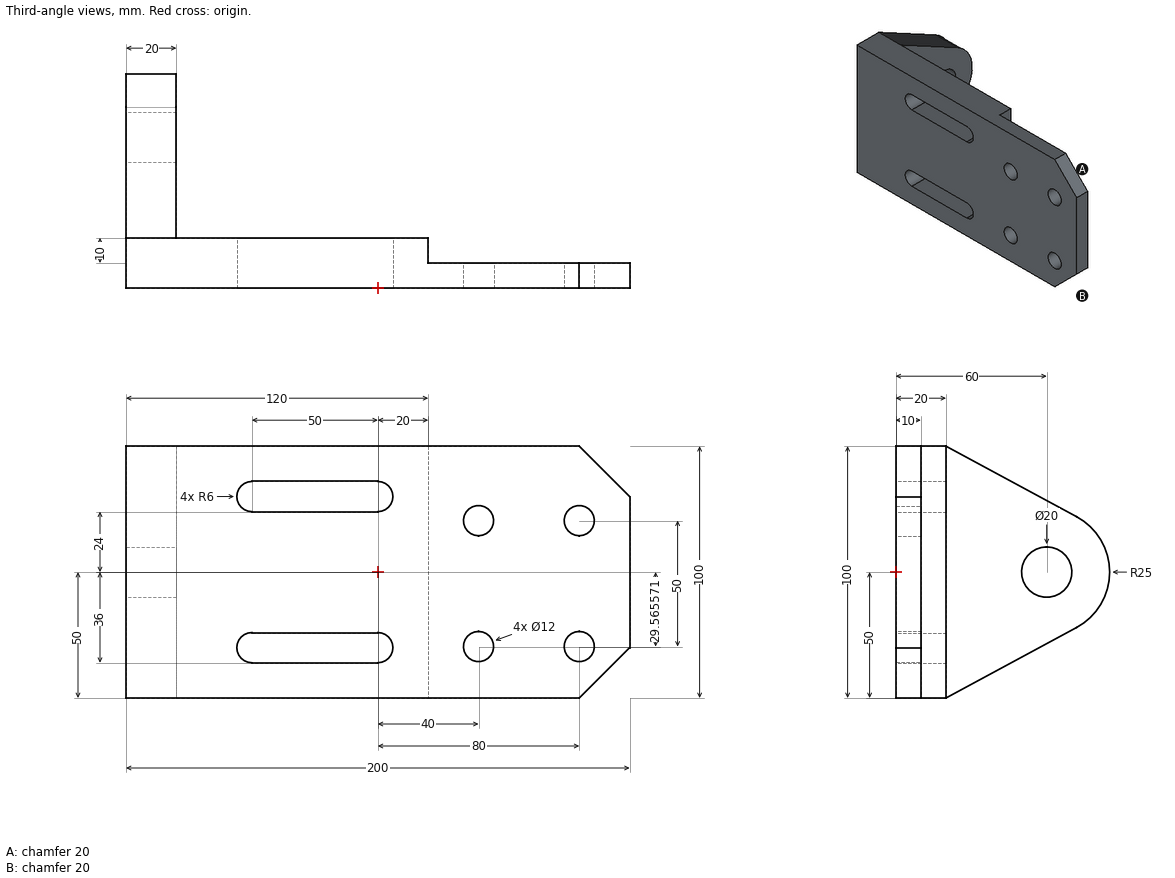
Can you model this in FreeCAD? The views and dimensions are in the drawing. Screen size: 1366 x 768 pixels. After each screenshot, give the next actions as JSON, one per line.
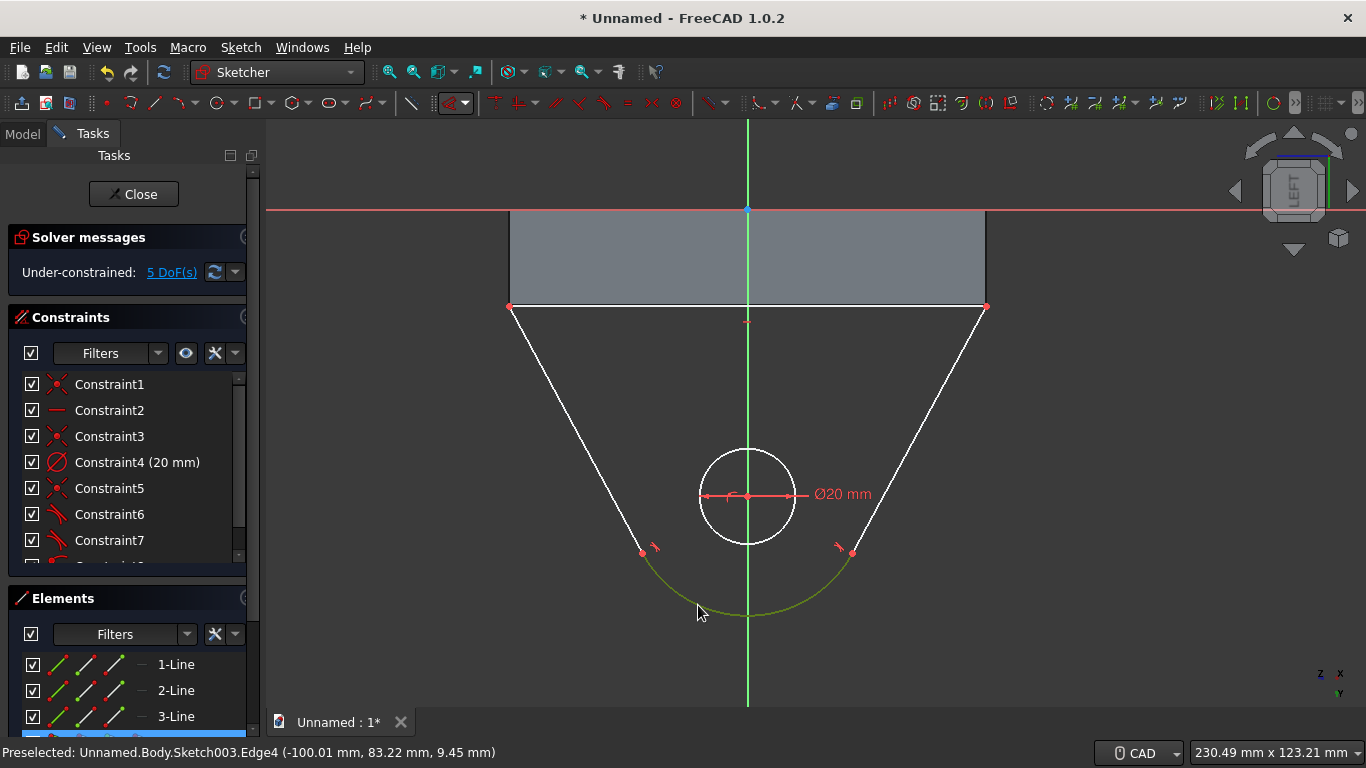
{"action": "key", "text": "k r"}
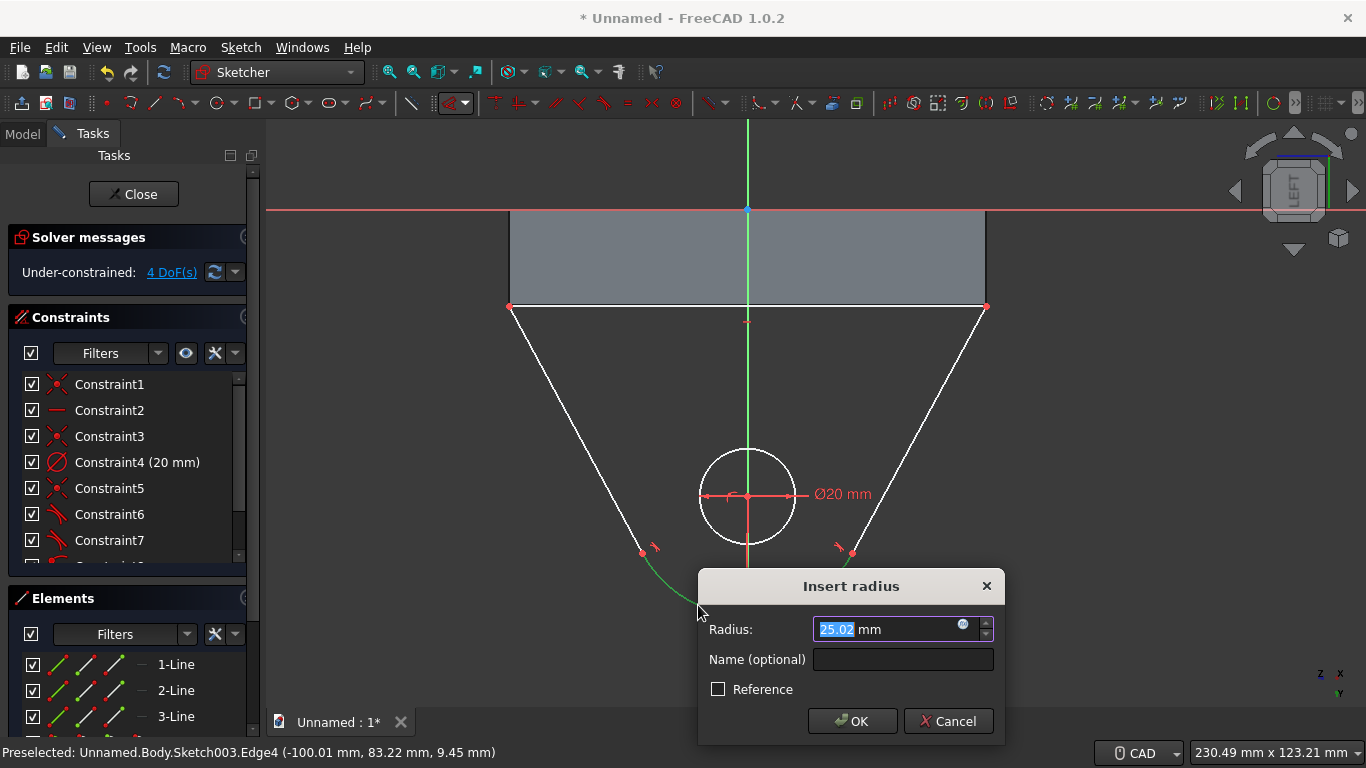
{"action": "type", "text": "25"}
{"action": "key", "text": "Return"}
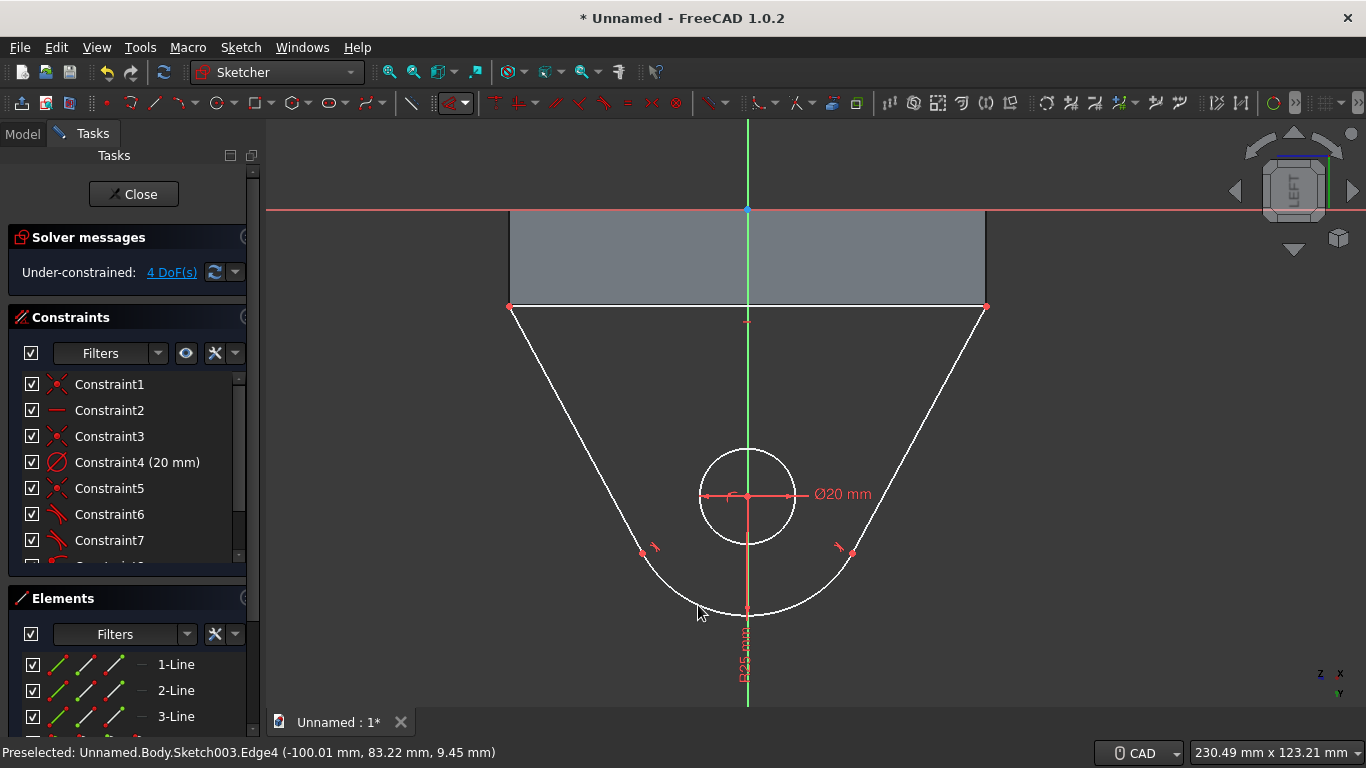
{"action": "left_click", "coordinate": [748, 496]}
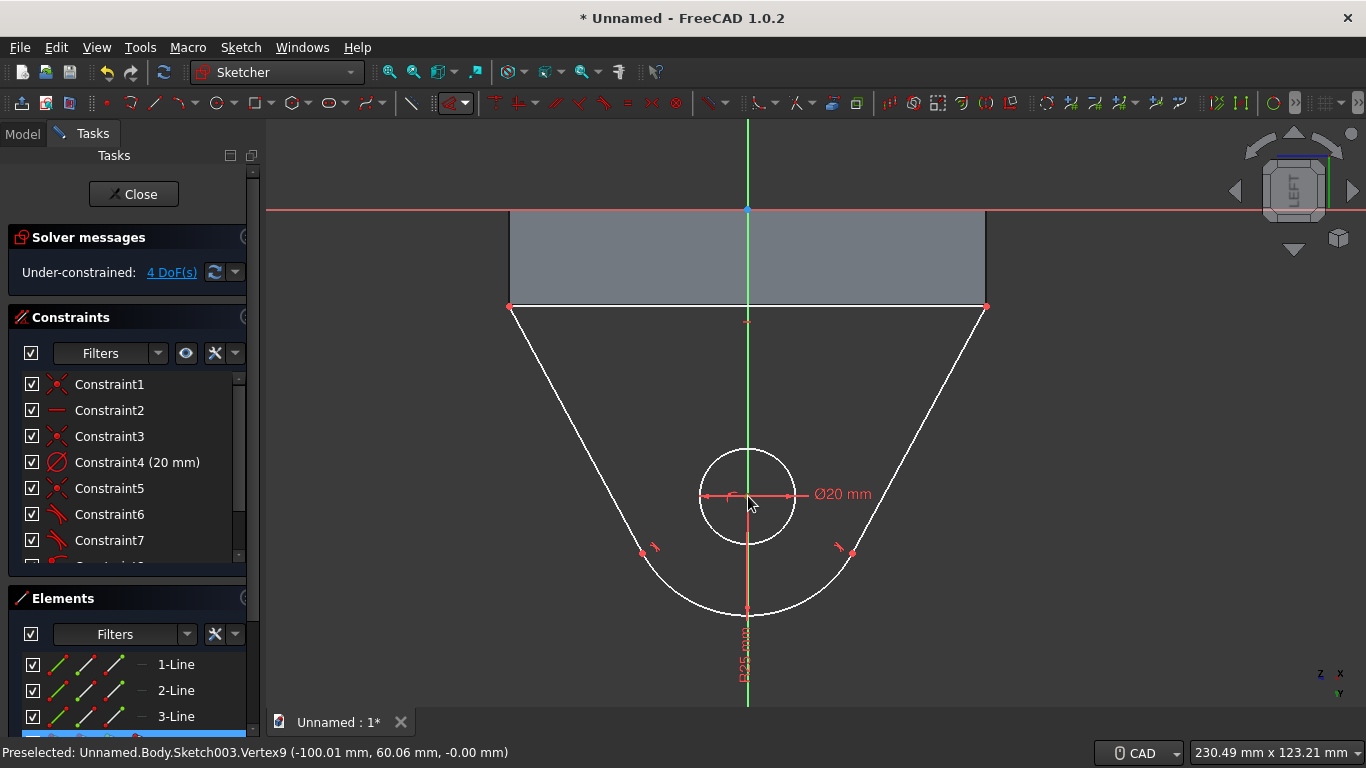
{"action": "key", "text": "i"}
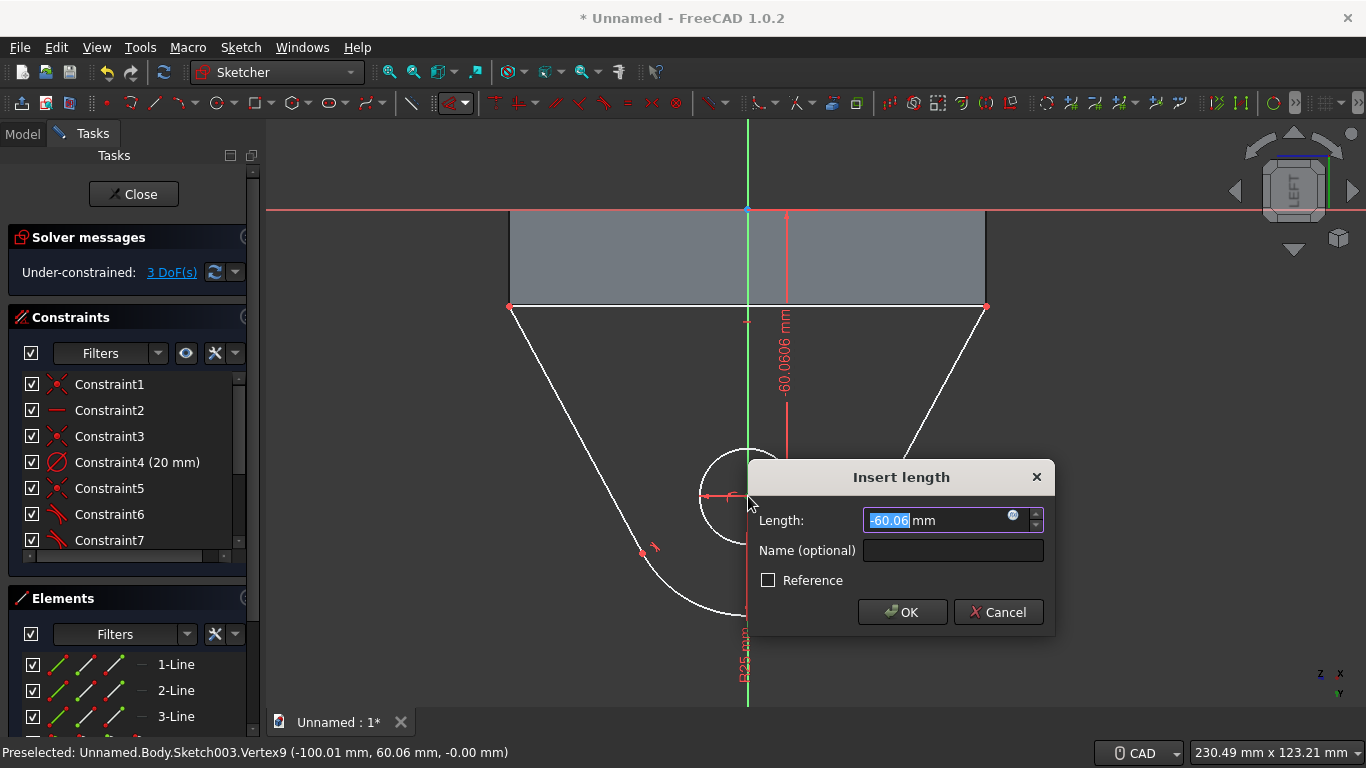
{"action": "type", "text": "-60"}
{"action": "key", "text": "Return"}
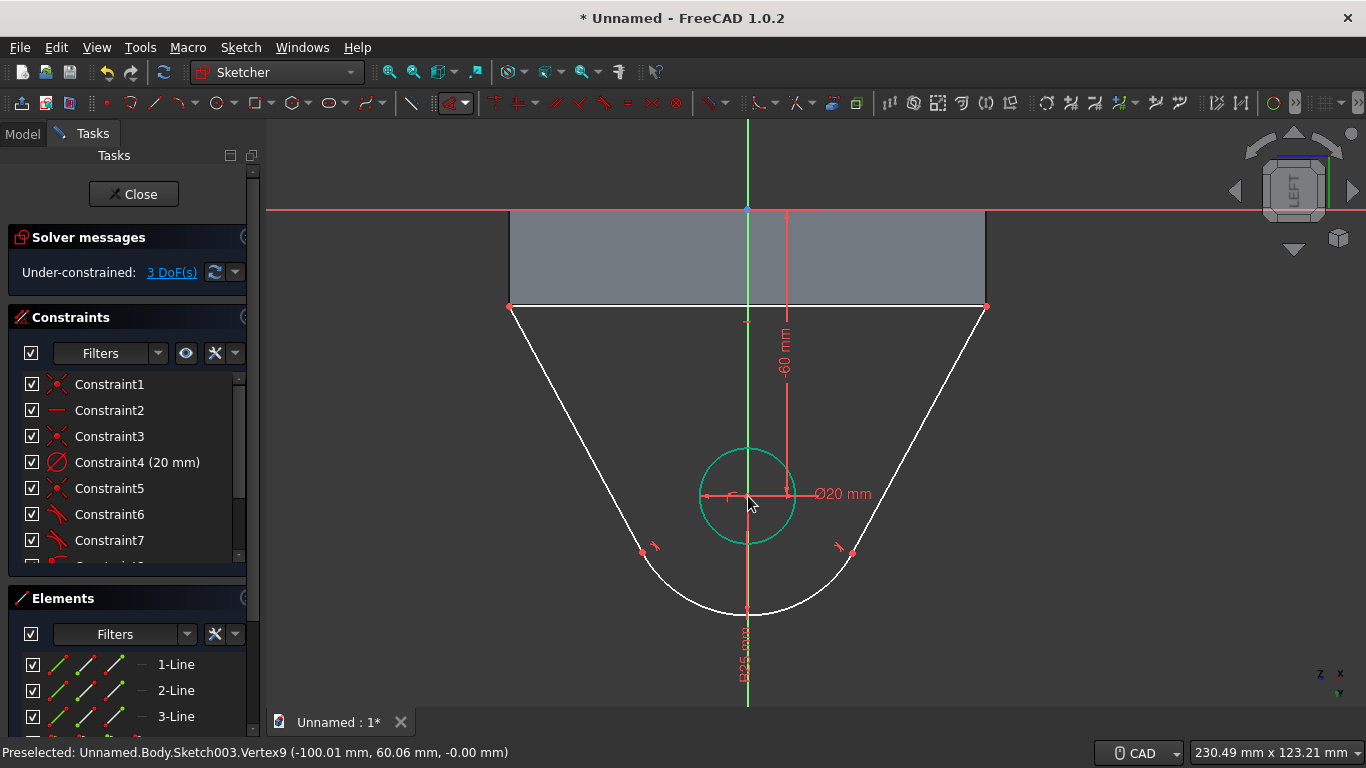
{"action": "left_click", "coordinate": [843, 306]}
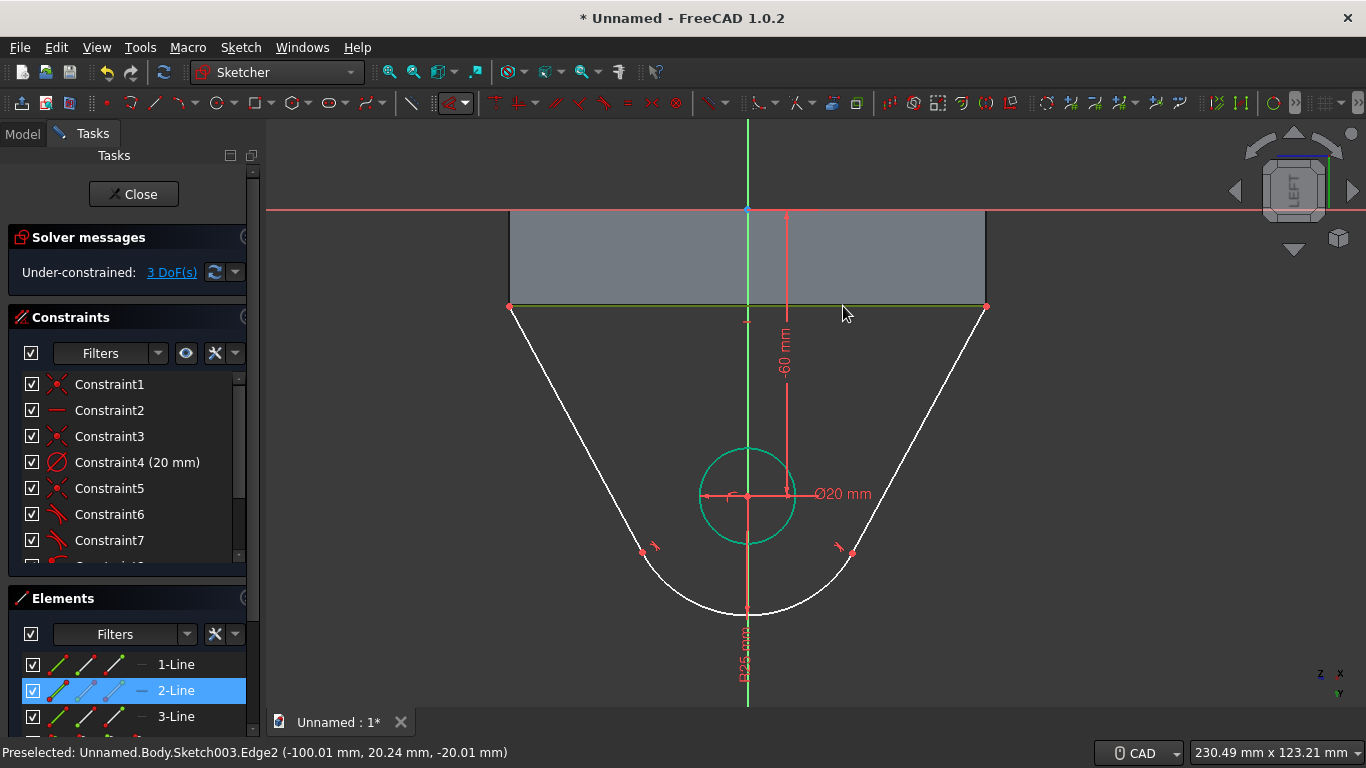
{"action": "left_click", "coordinate": [468, 104]}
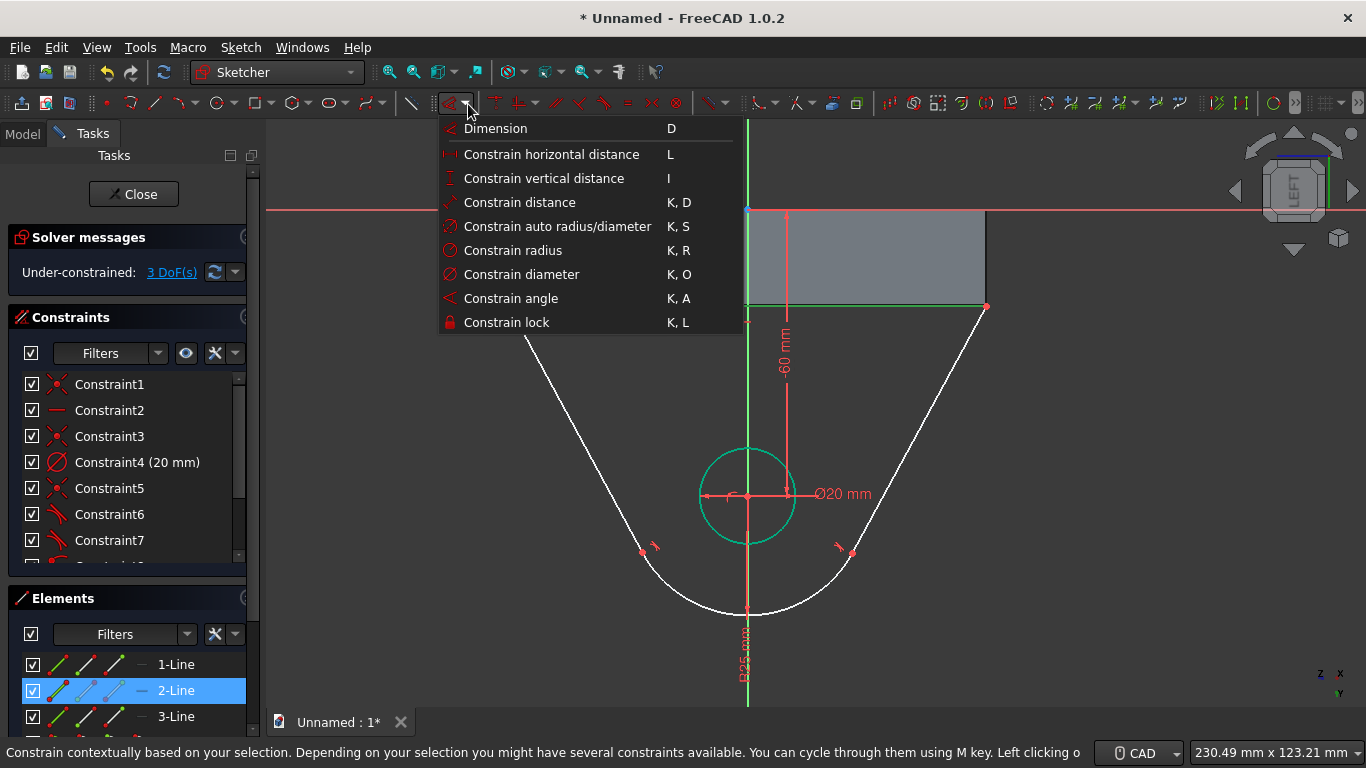
{"action": "left_click", "coordinate": [591, 154]}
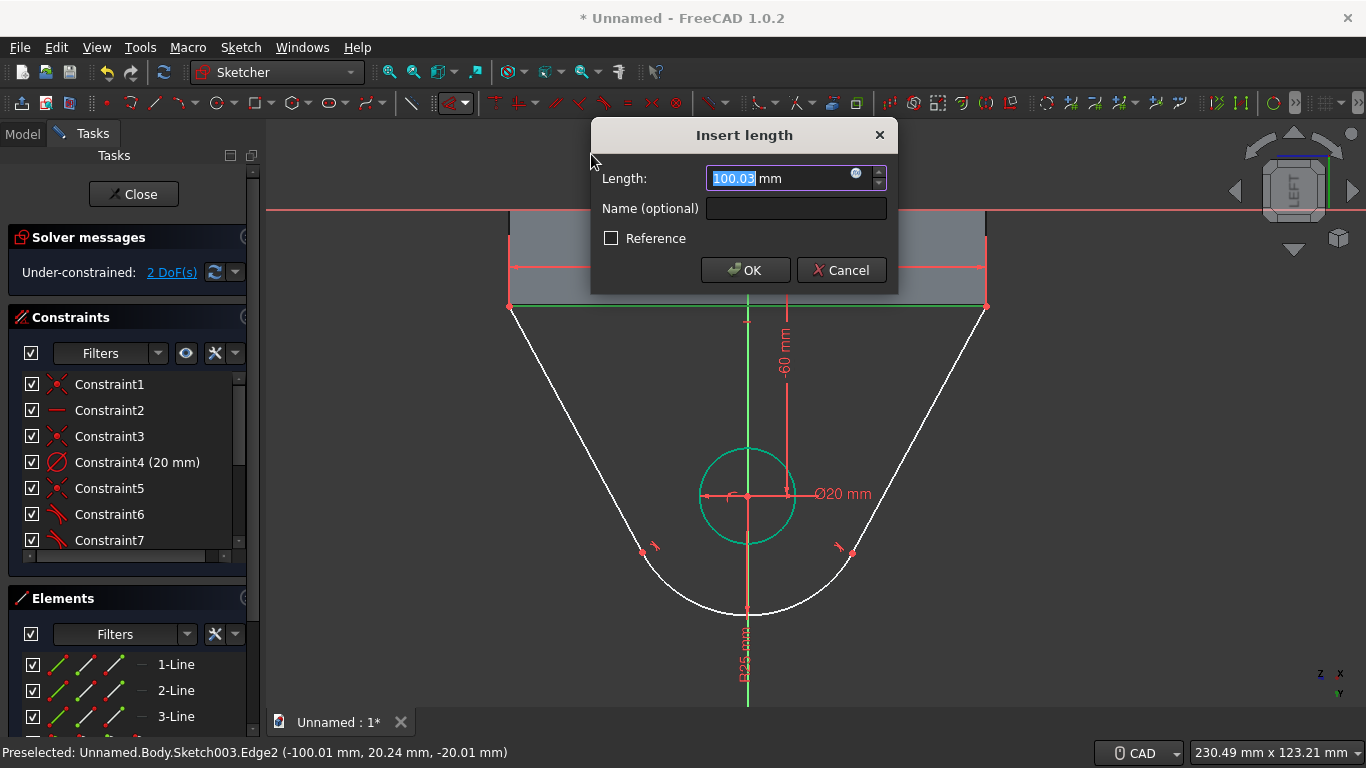
{"action": "type", "text": "100"}
{"action": "key", "text": "Return"}